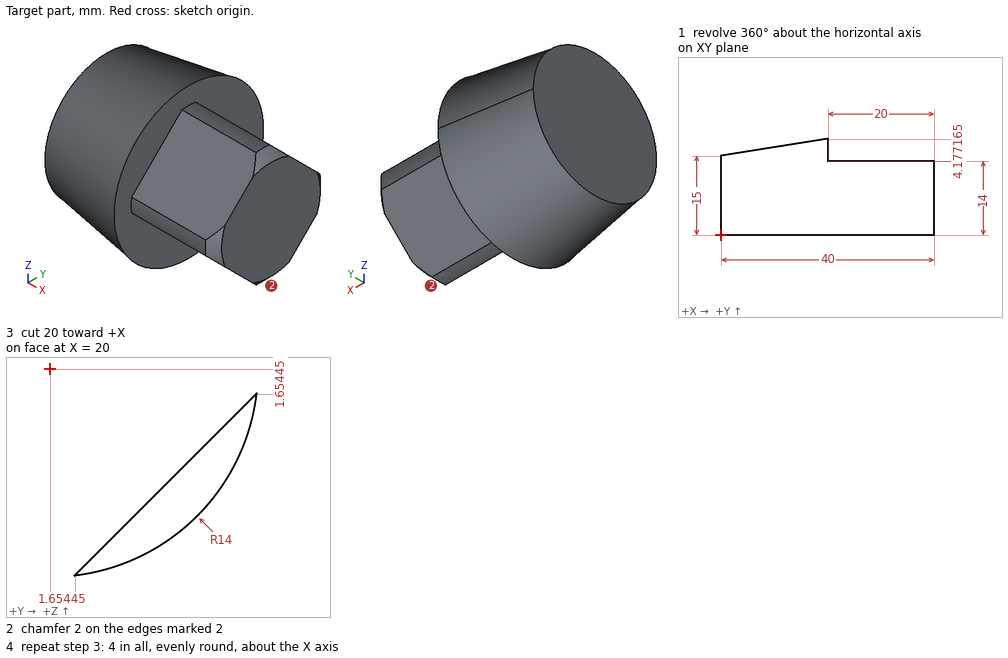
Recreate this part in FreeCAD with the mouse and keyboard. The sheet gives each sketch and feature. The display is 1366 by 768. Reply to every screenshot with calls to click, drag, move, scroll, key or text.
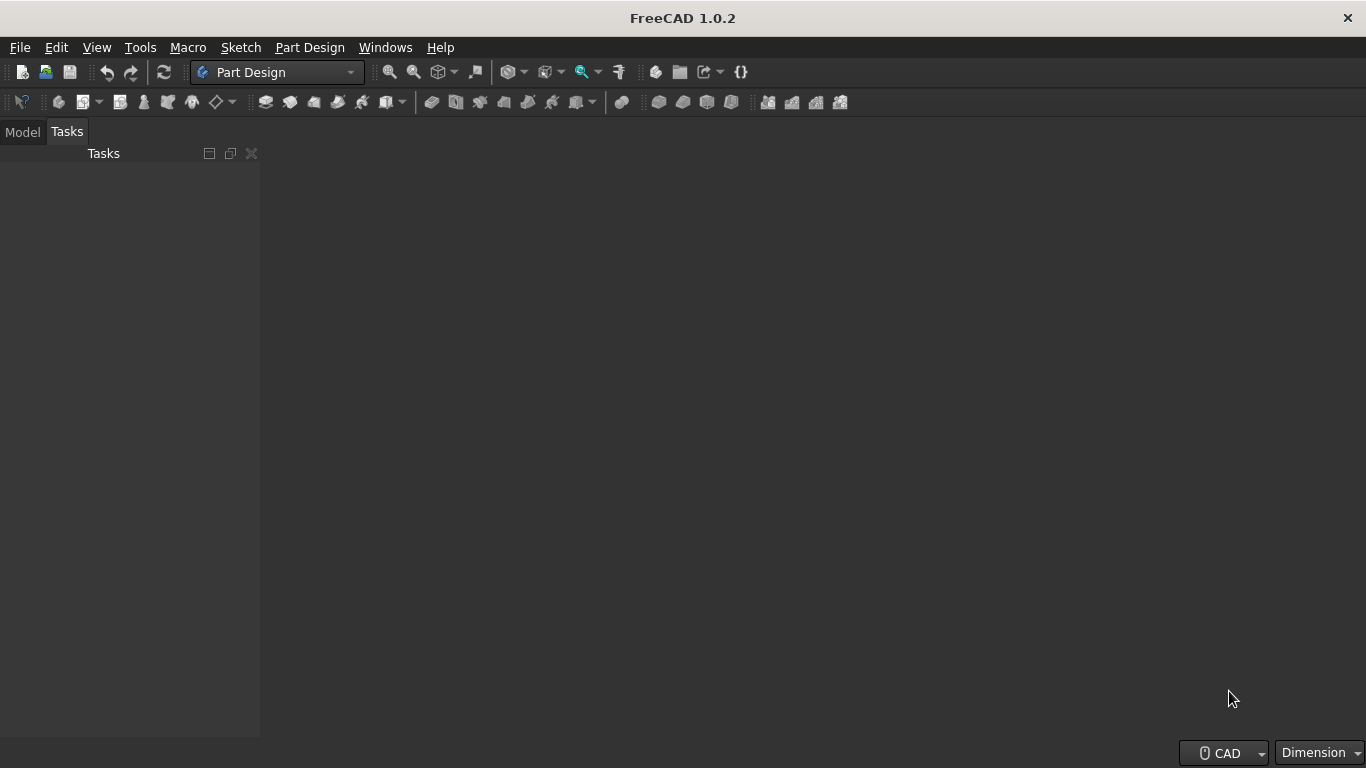
key(ctrl+n)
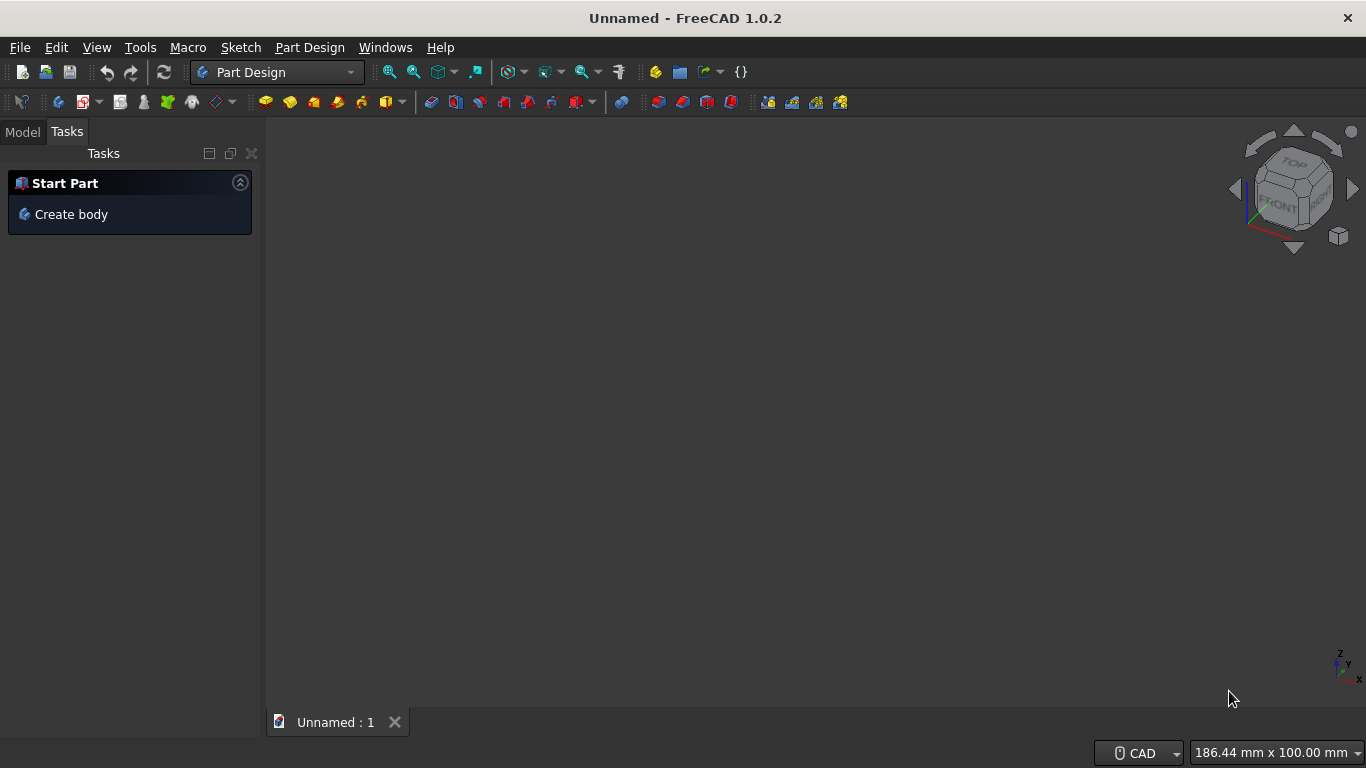
click(84, 102)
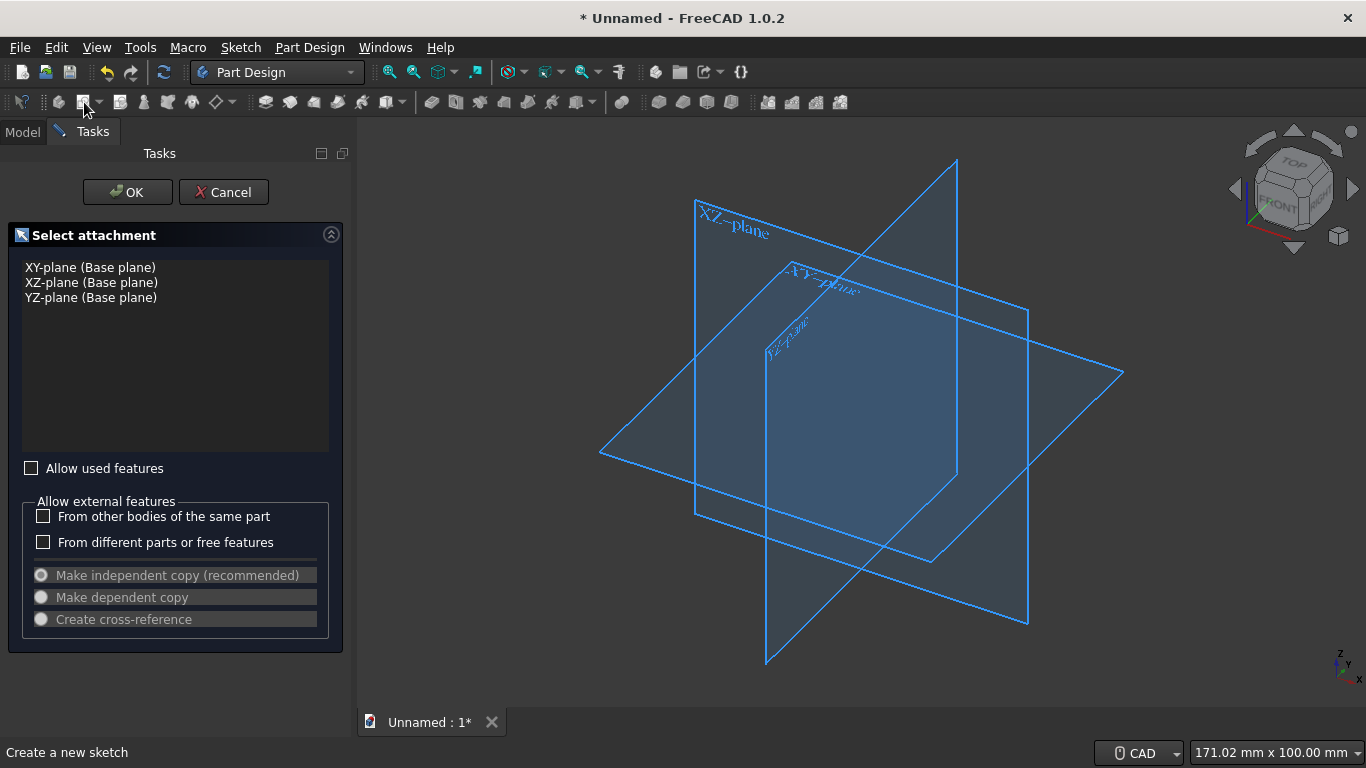
click(82, 268)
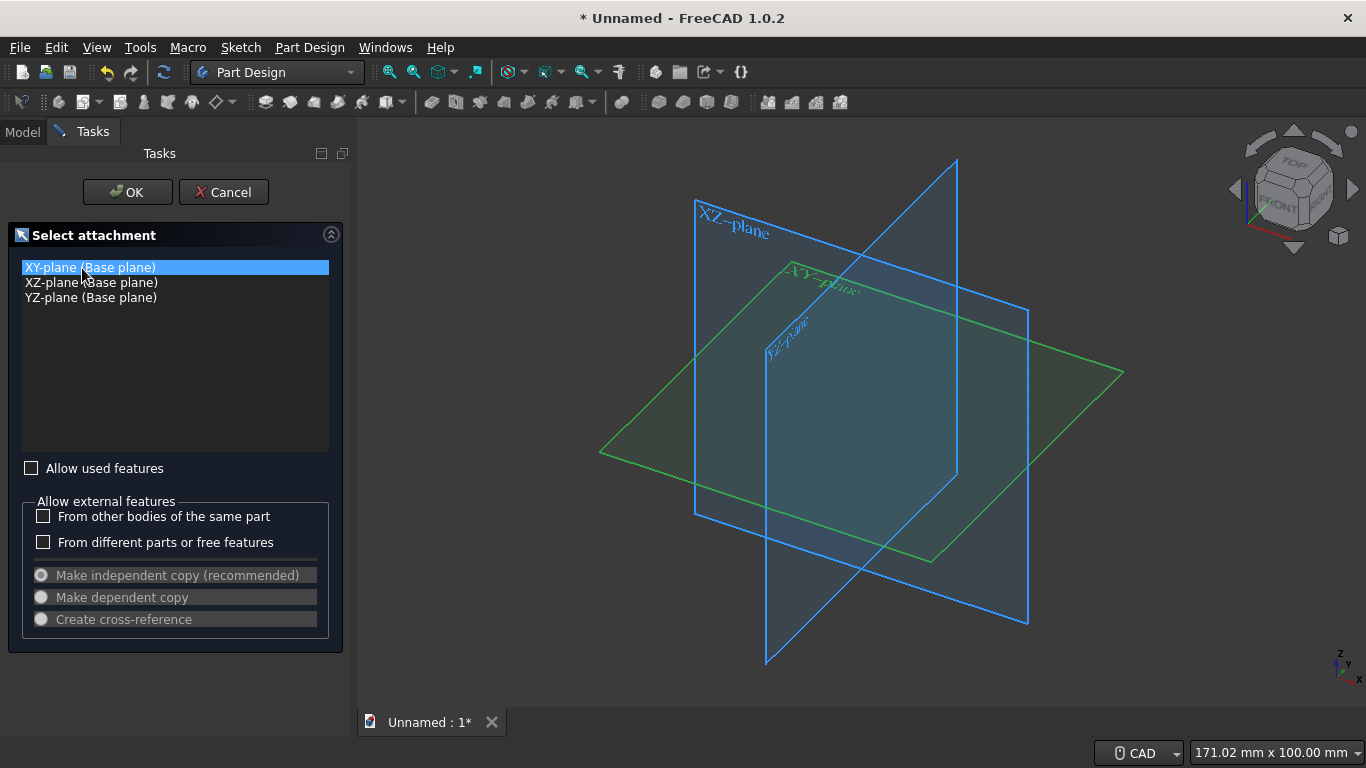
click(128, 192)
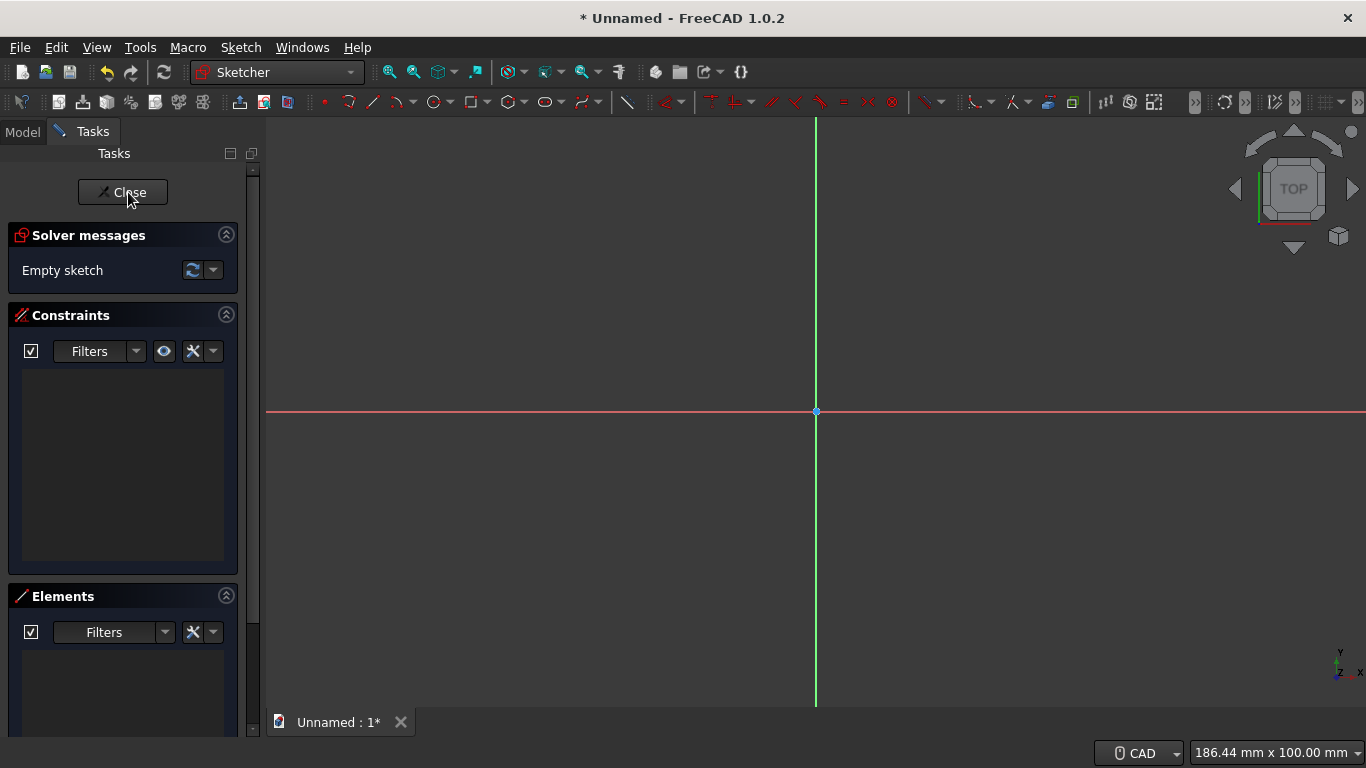
scroll(1043, 327, up, 5)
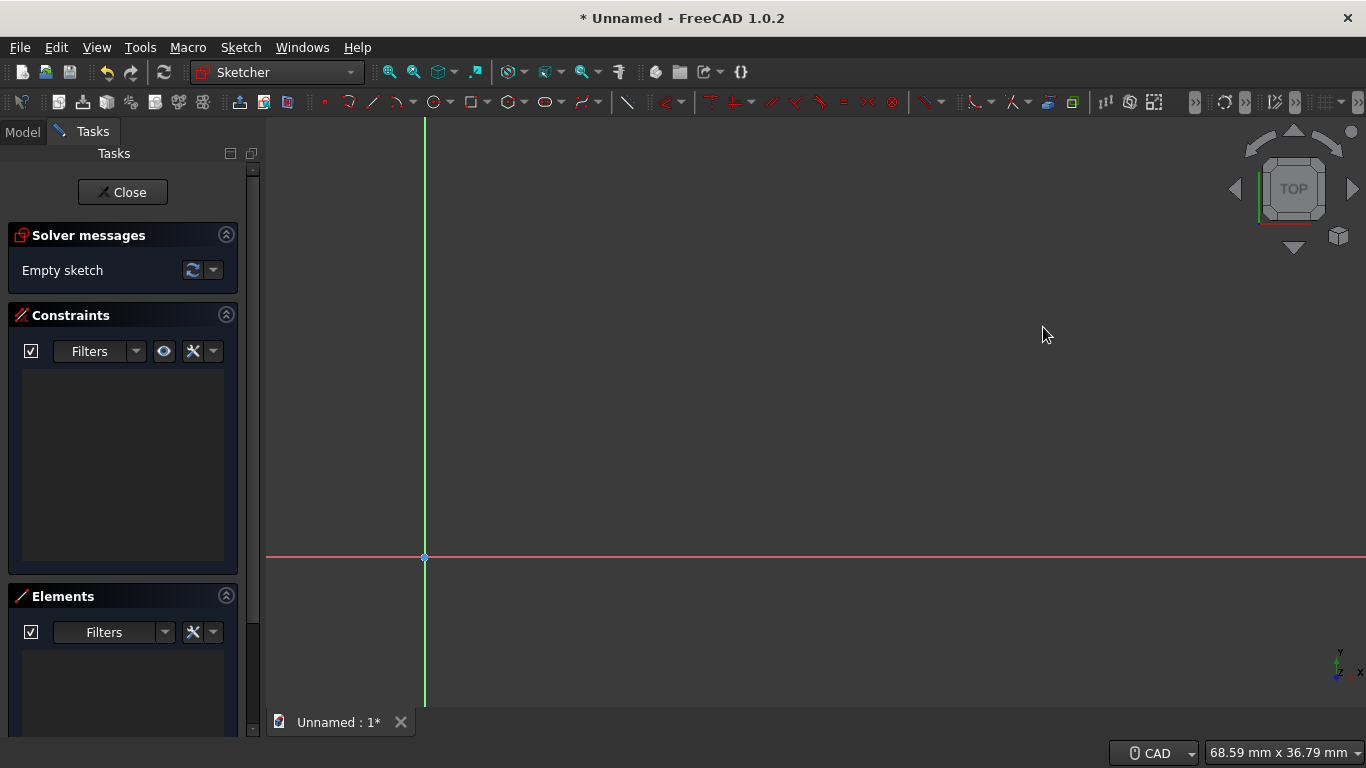
key(g)
key(m)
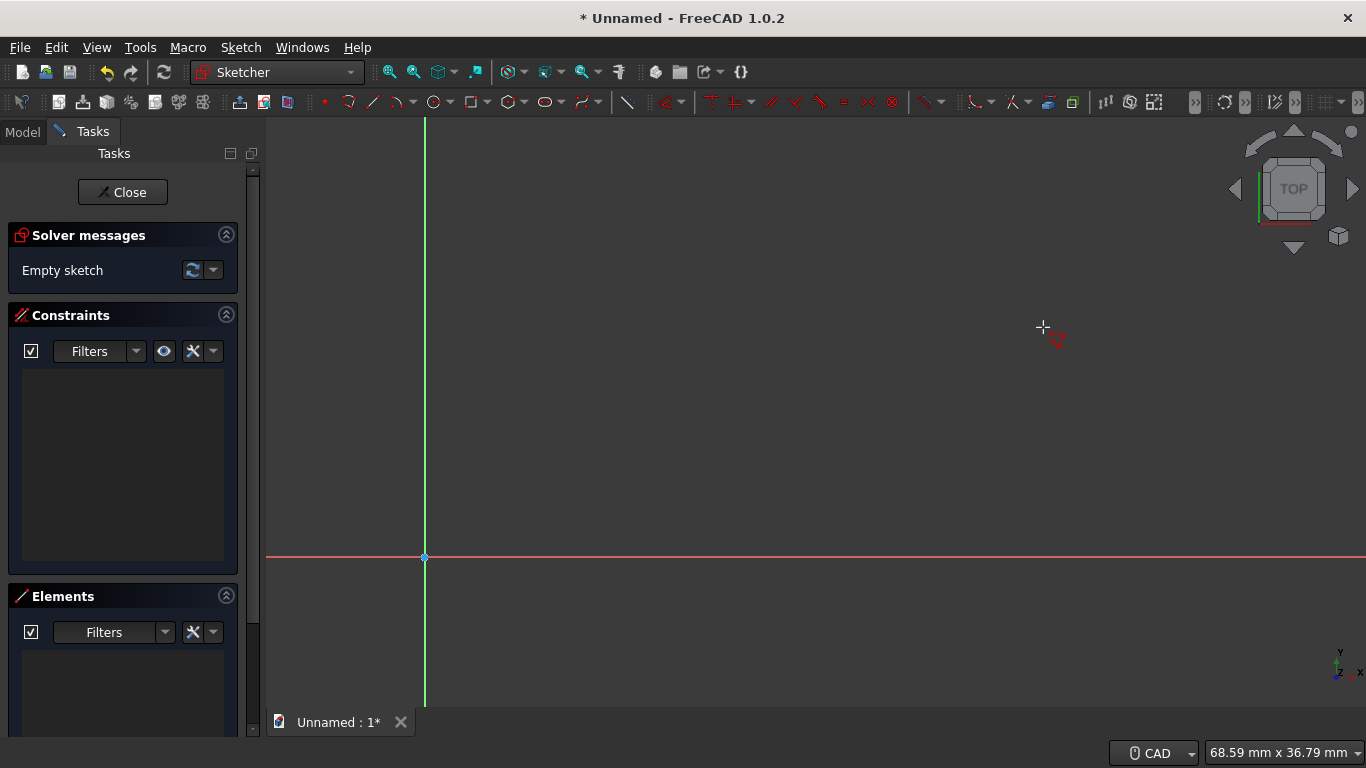
click(425, 557)
click(1066, 548)
click(1066, 333)
click(745, 333)
click(745, 266)
click(434, 317)
click(425, 557)
key(Escape)
key(Escape)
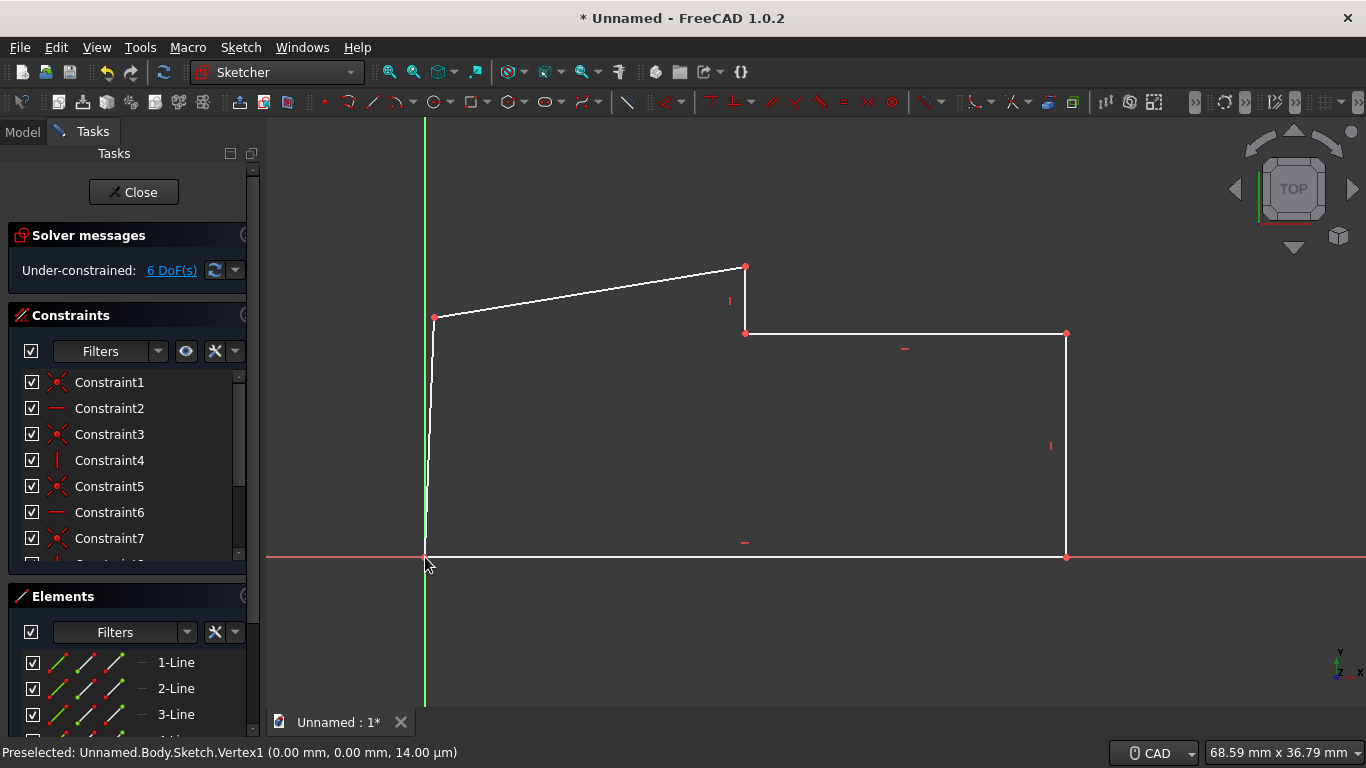
click(428, 486)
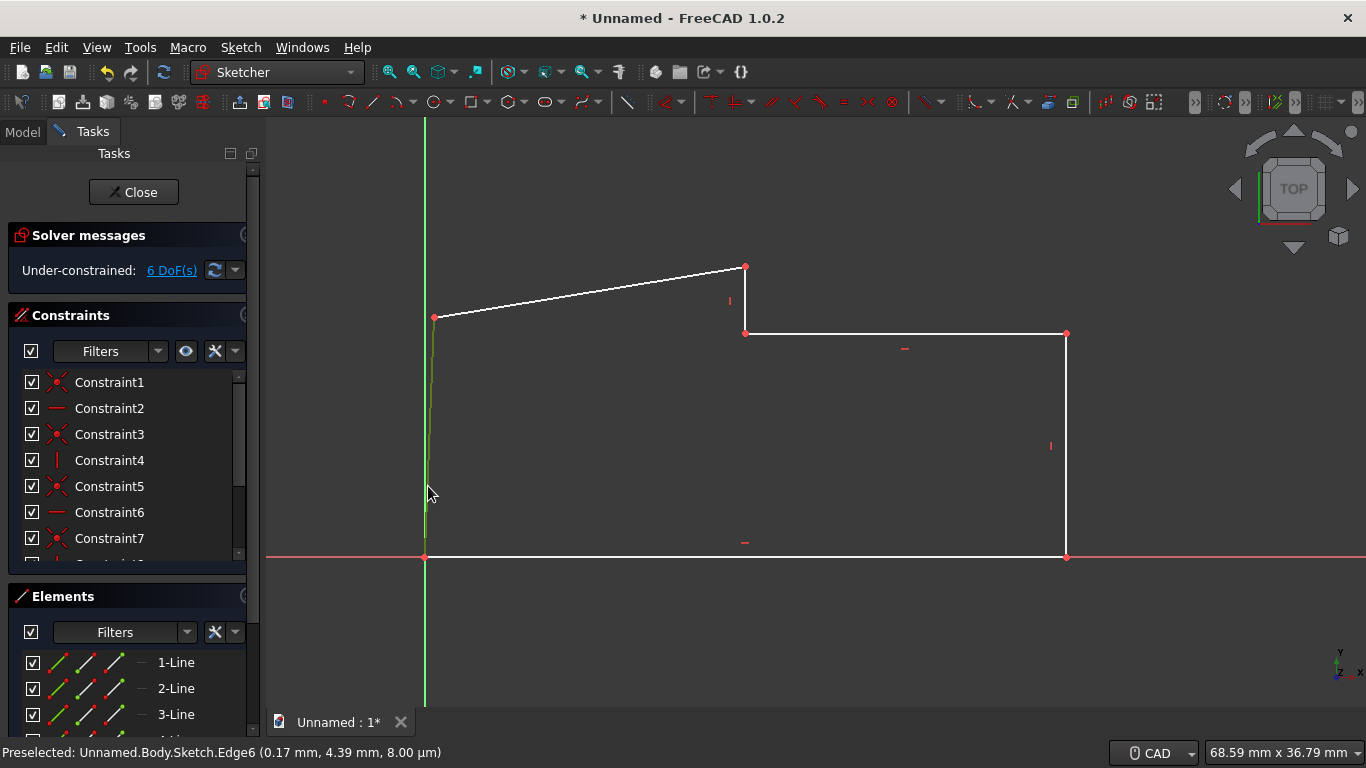
key(v)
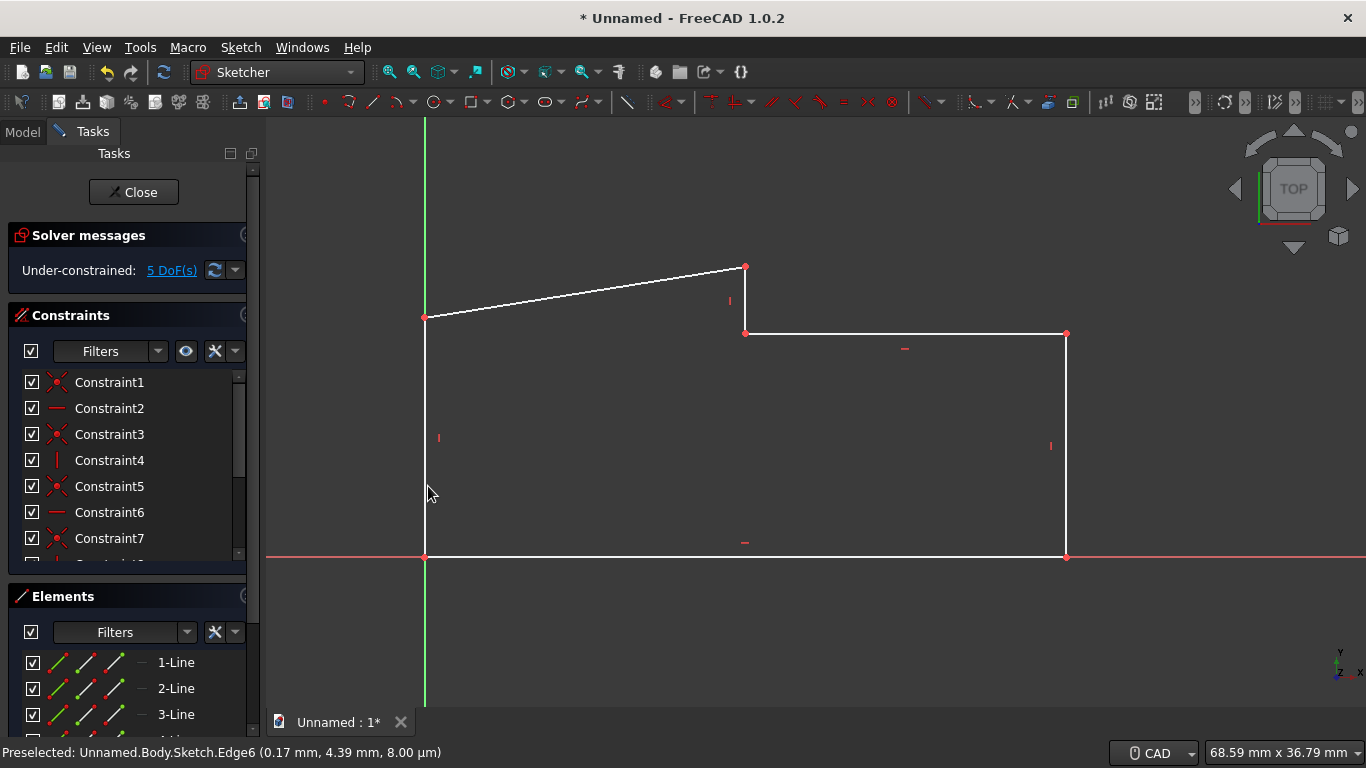
key(d)